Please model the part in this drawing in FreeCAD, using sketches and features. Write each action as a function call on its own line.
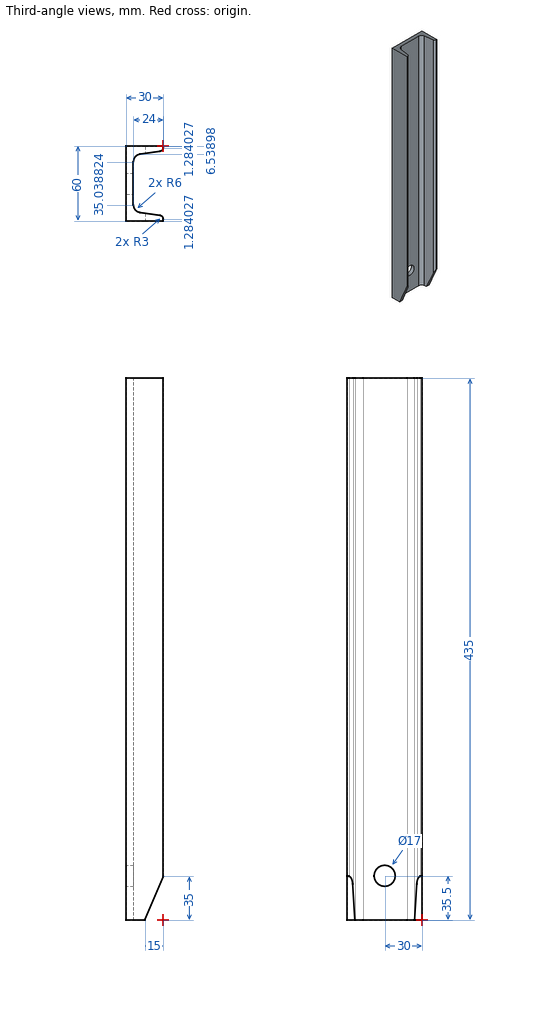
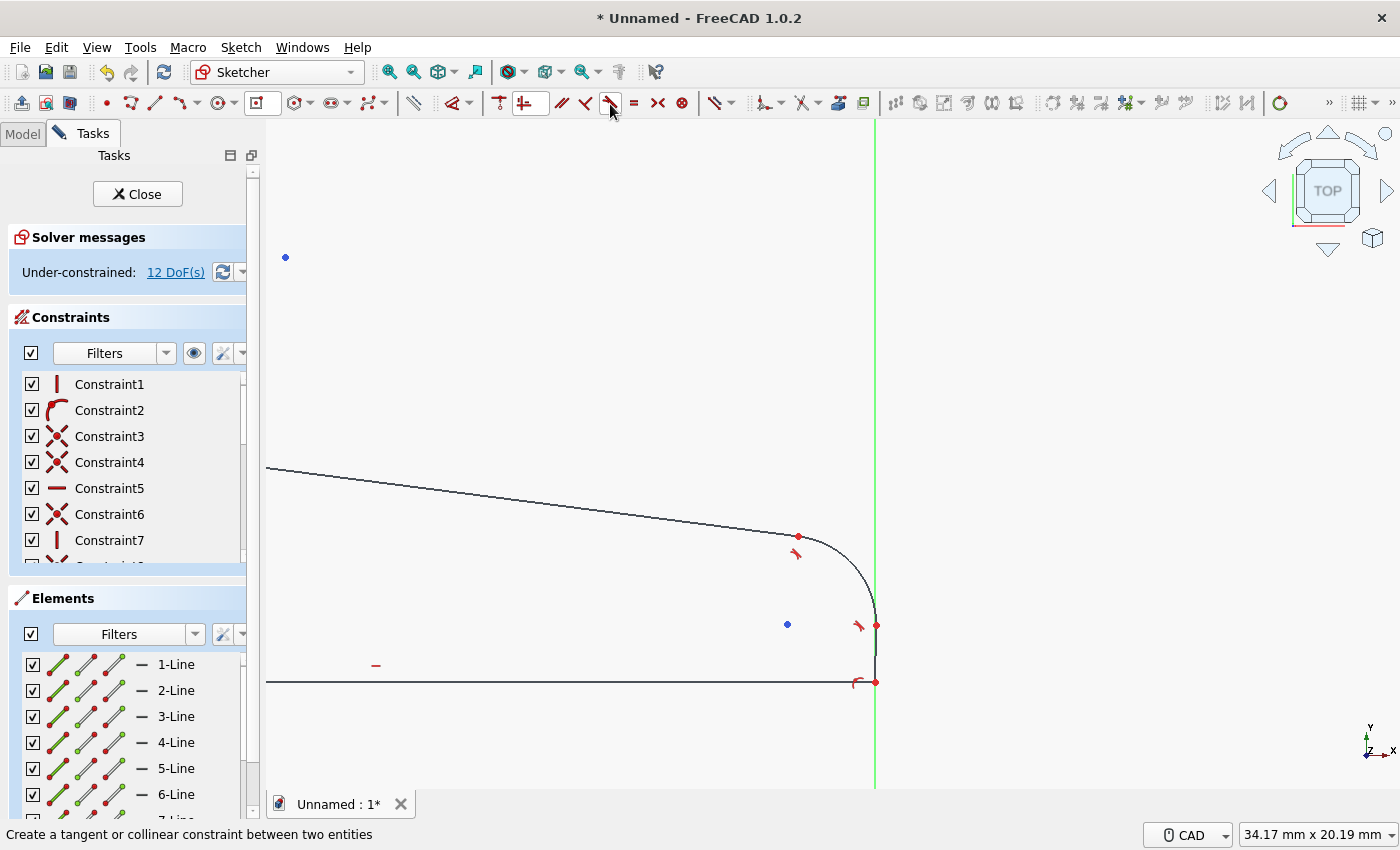
click(875, 665)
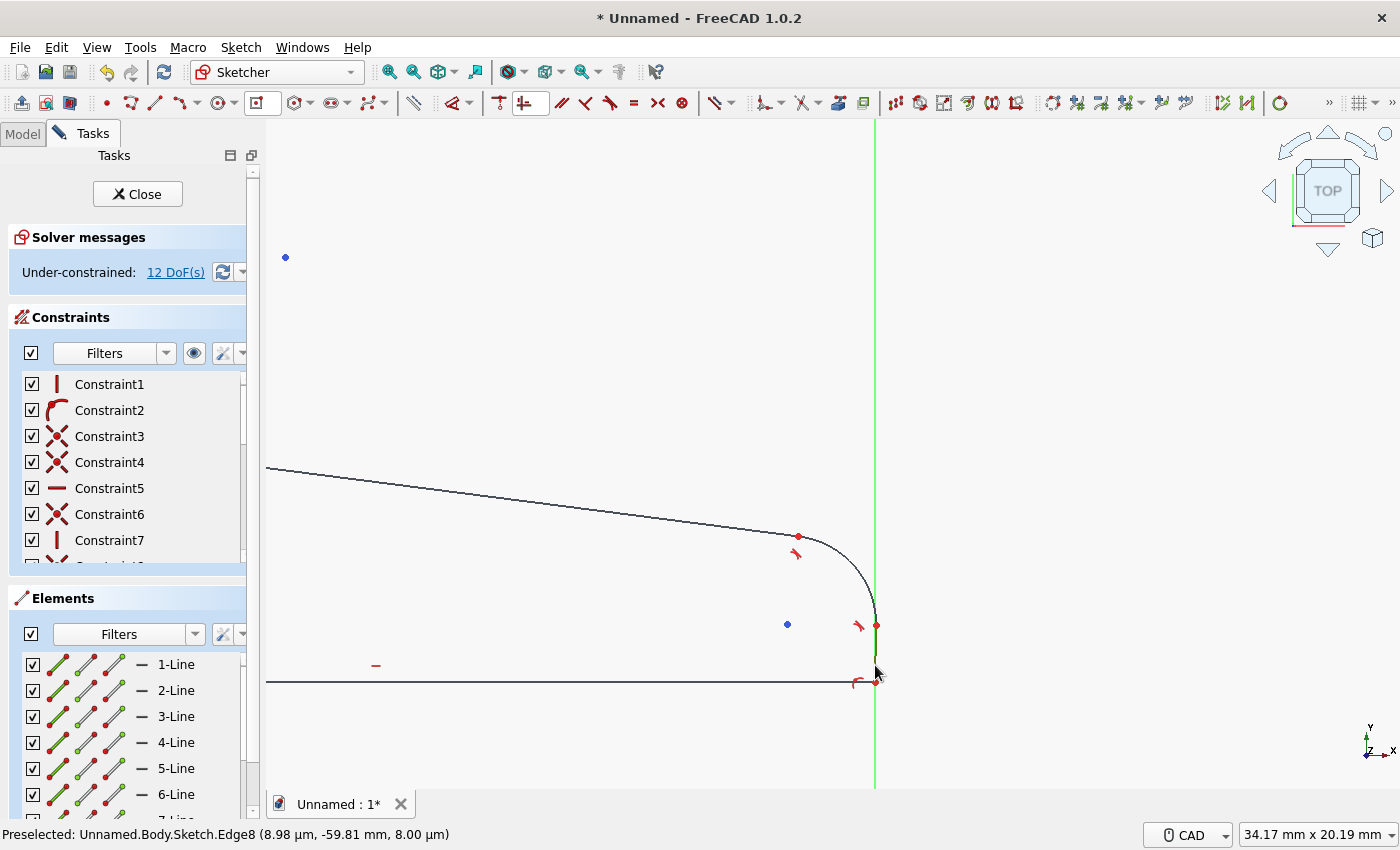
key(v)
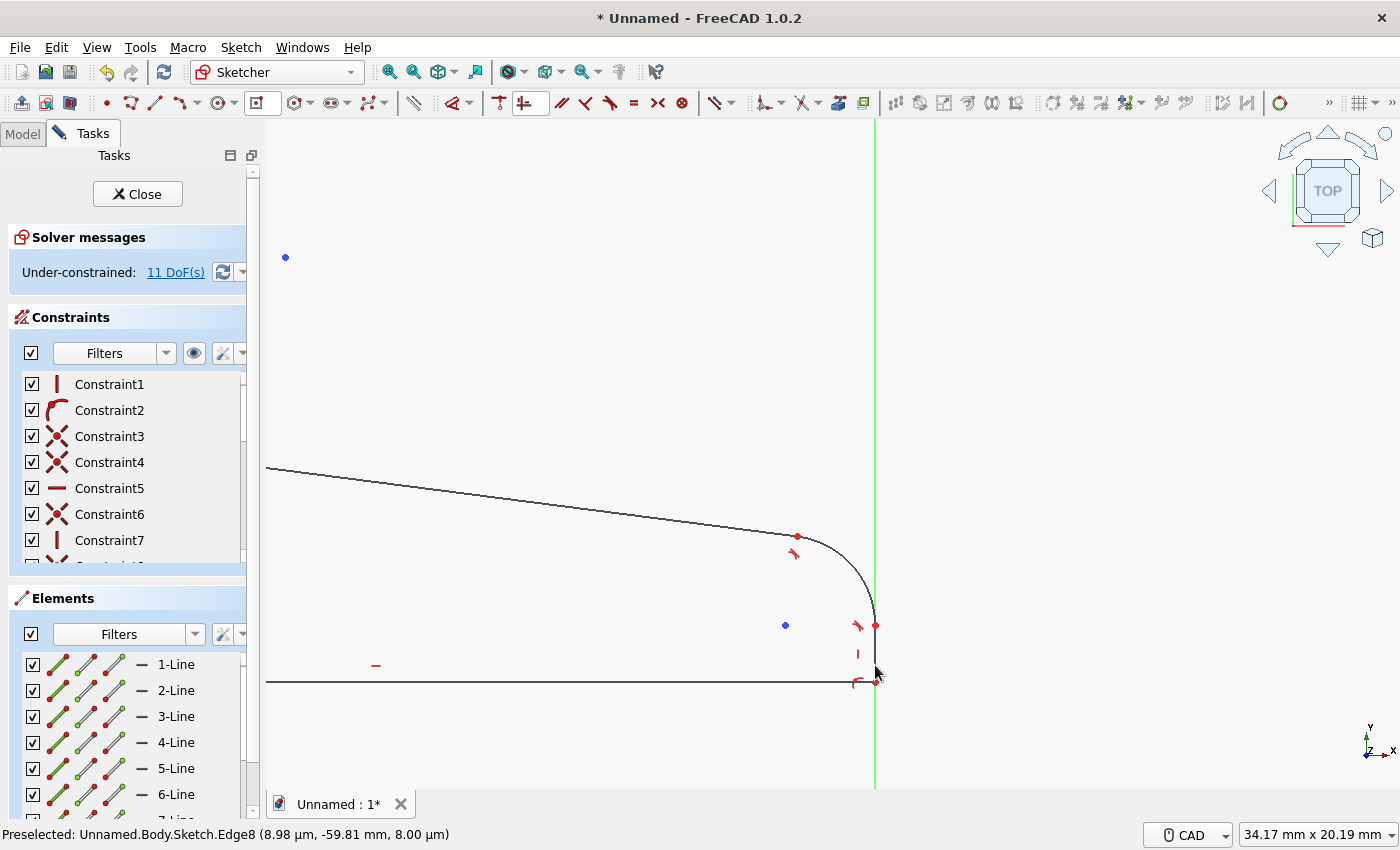
scroll(862, 651, down, 8)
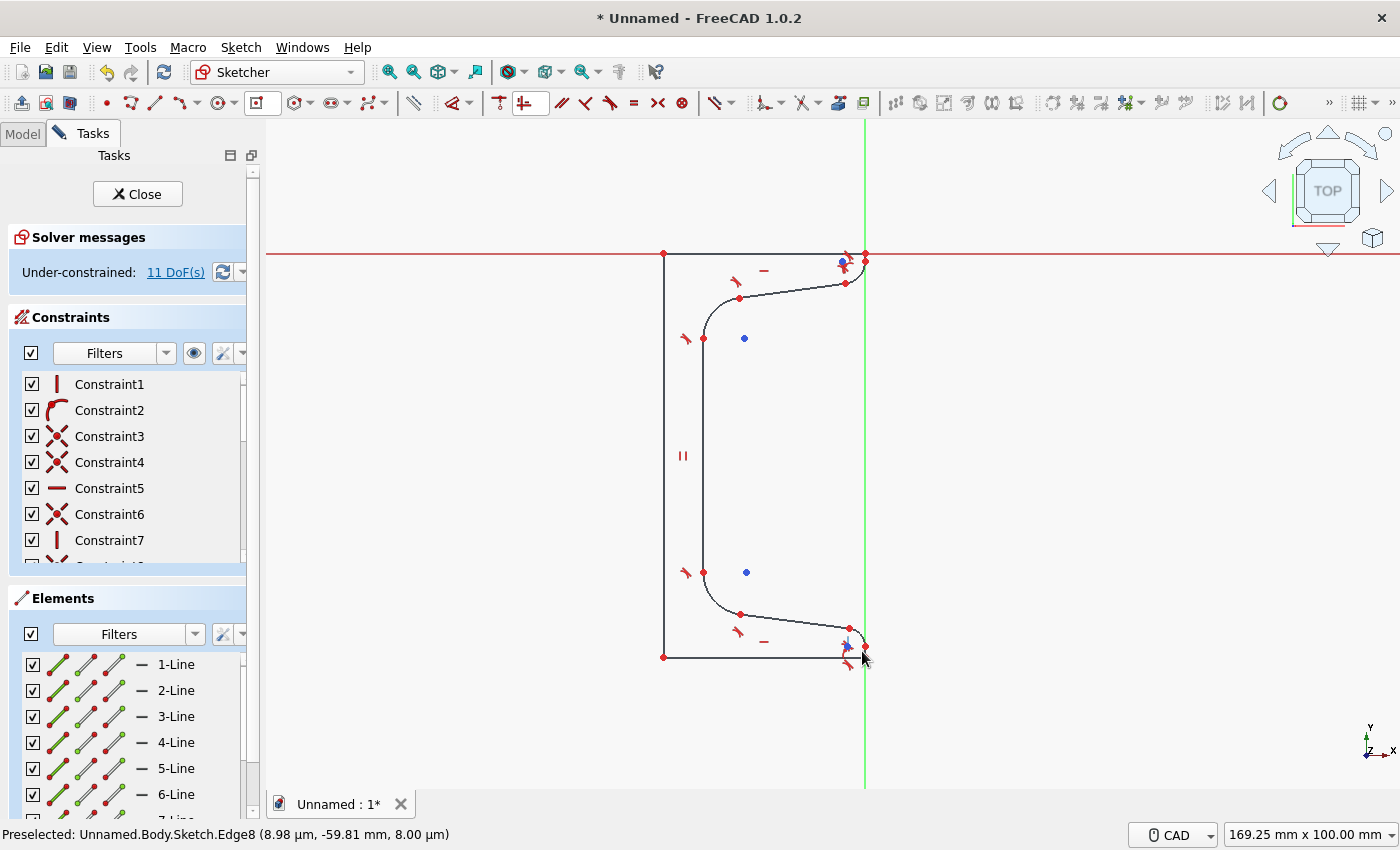
click(707, 590)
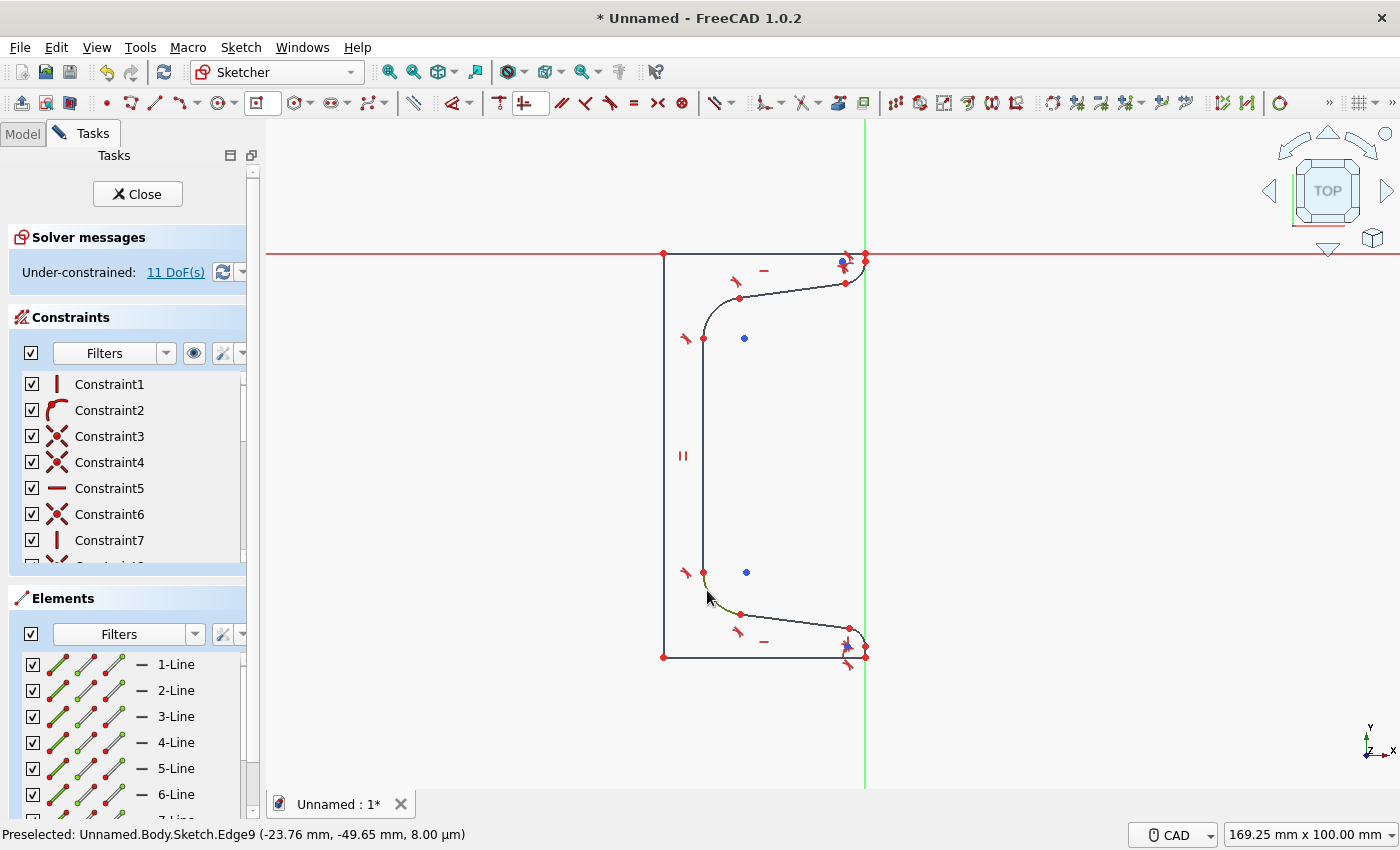
click(723, 304)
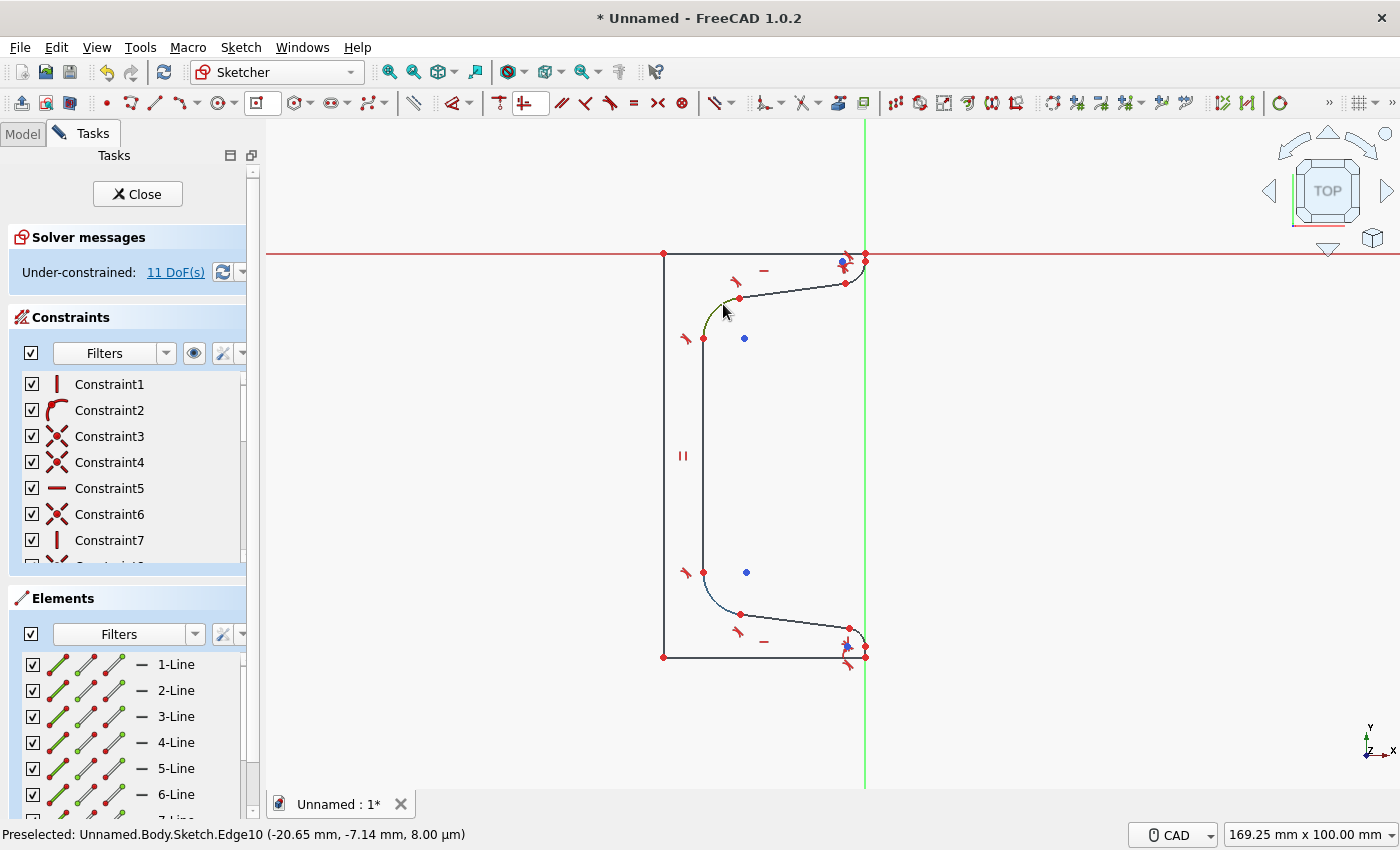
click(634, 104)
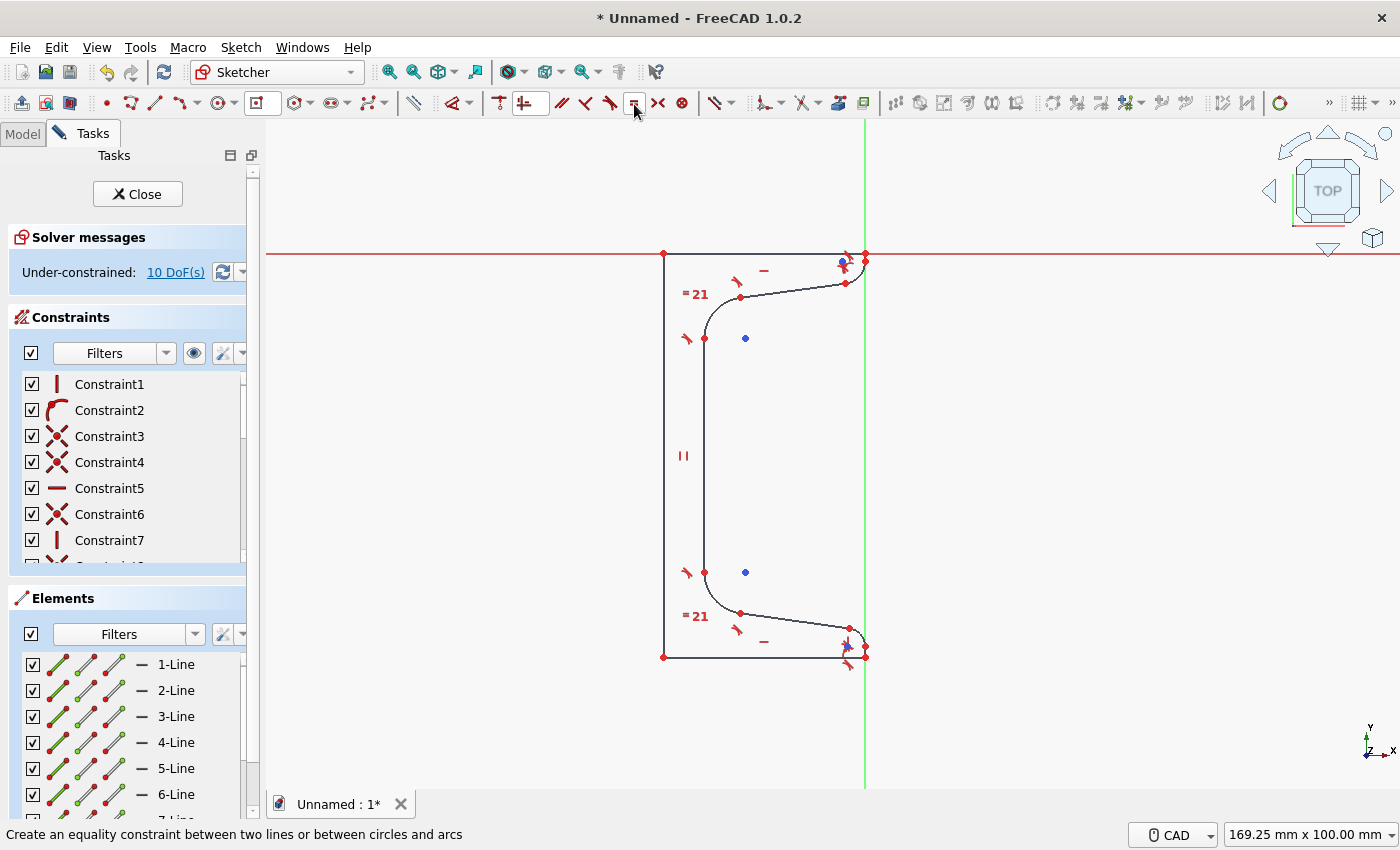
scroll(855, 280, up, 2)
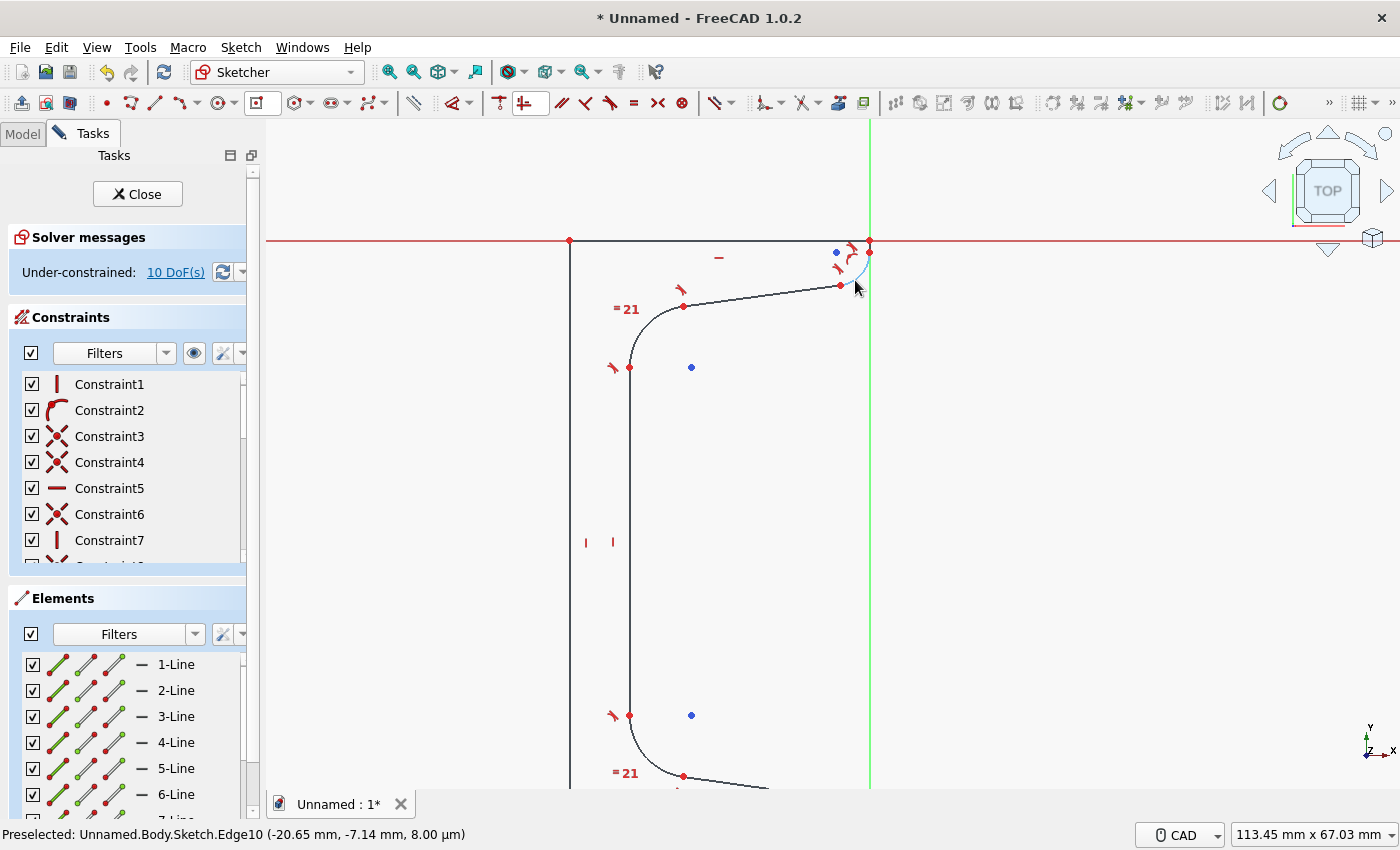
click(854, 280)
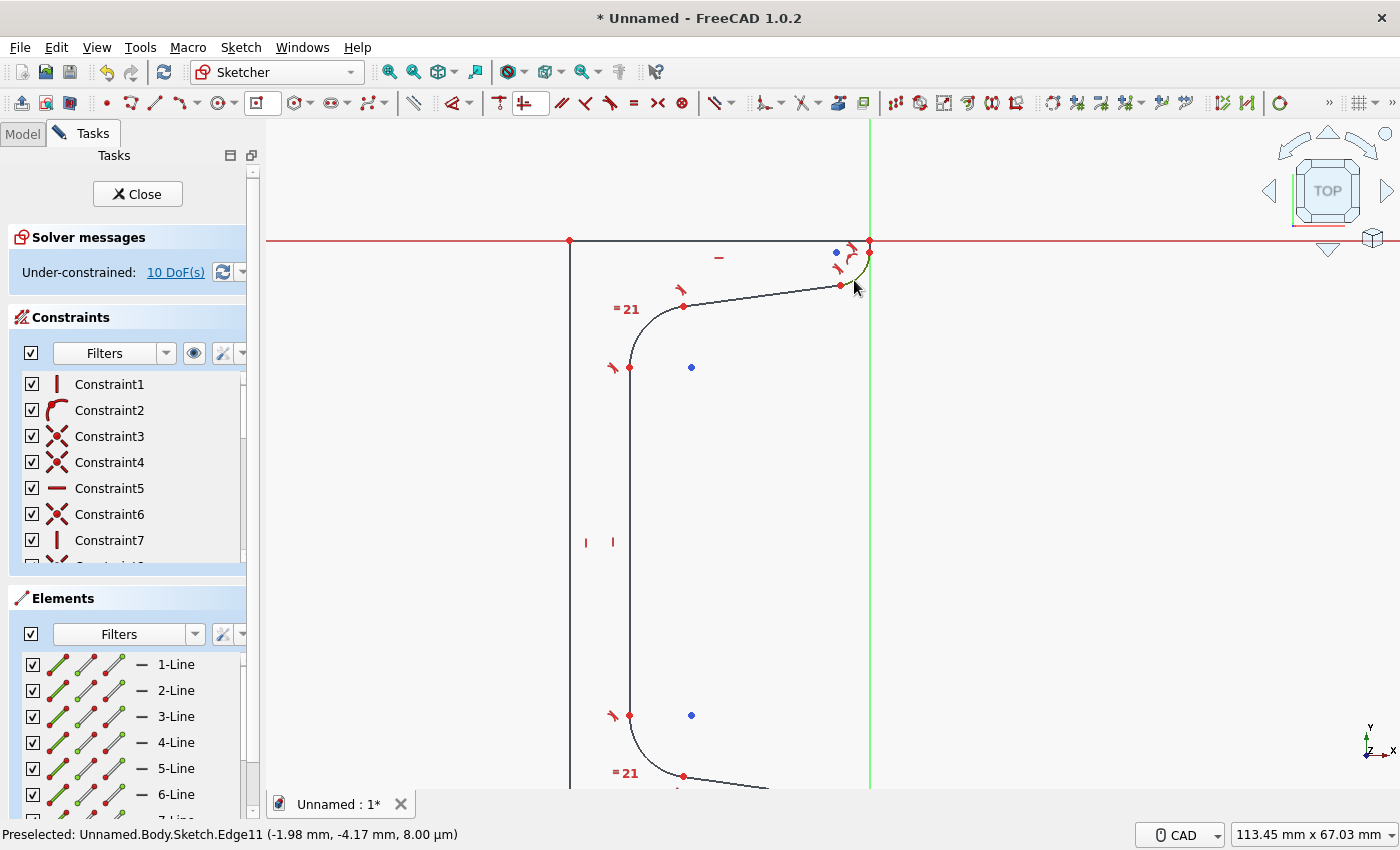
scroll(855, 277, down, 2)